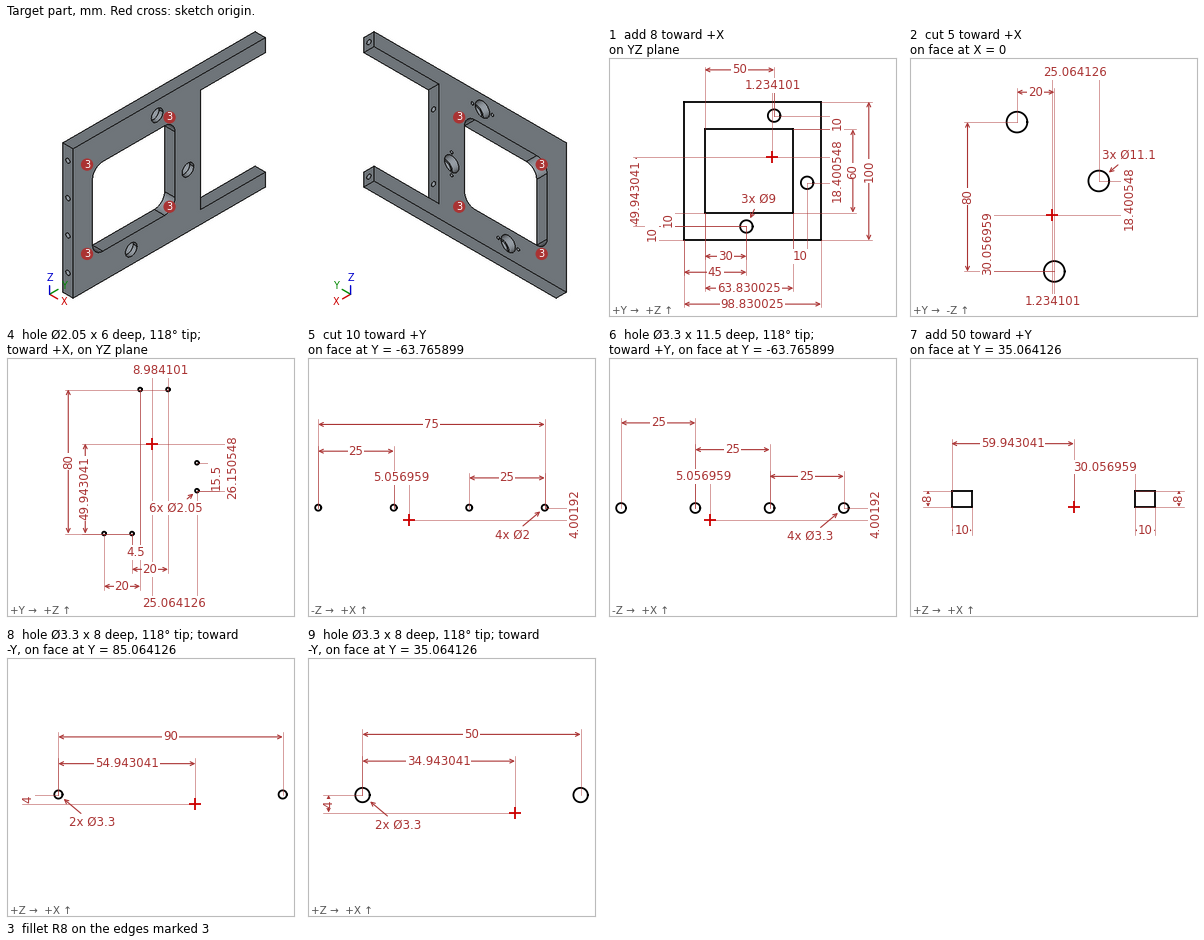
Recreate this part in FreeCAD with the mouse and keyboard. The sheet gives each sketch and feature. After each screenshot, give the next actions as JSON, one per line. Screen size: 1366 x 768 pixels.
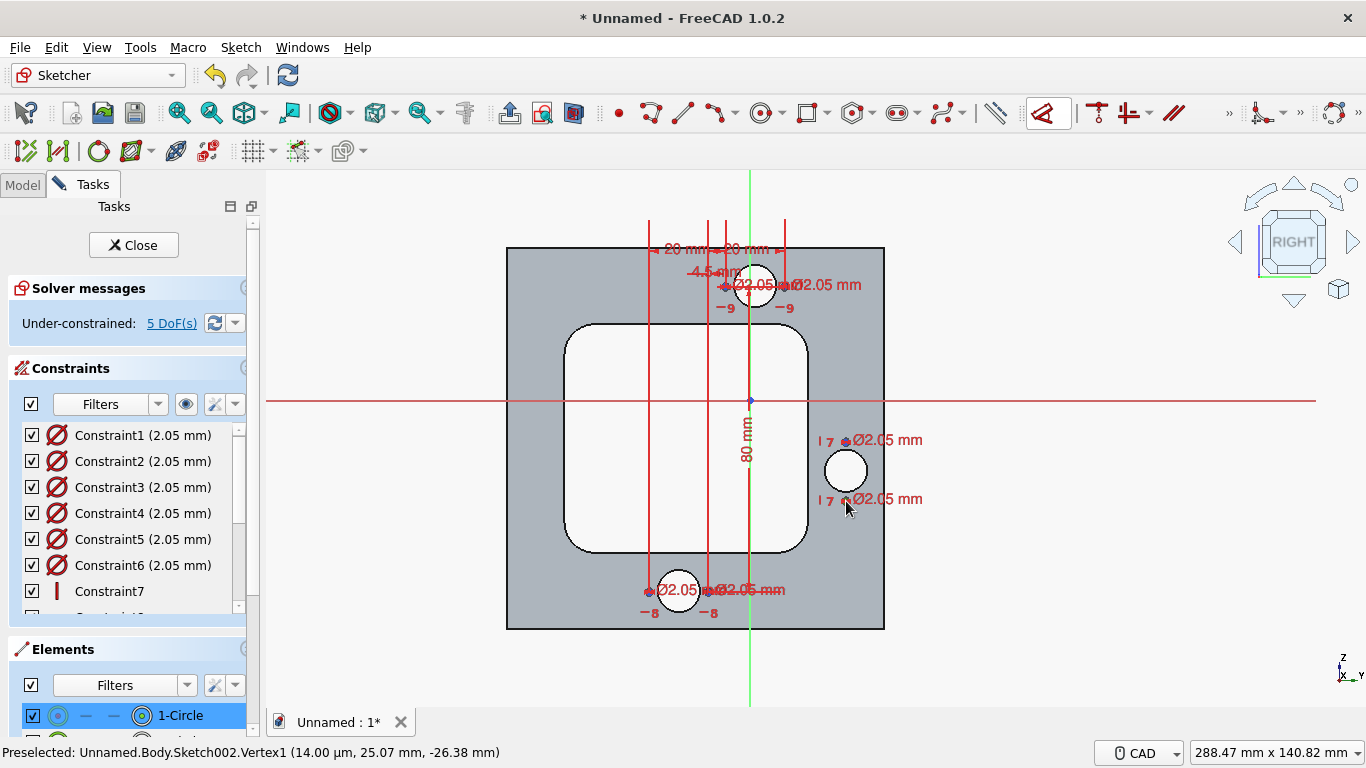
{"action": "left_click", "coordinate": [846, 442]}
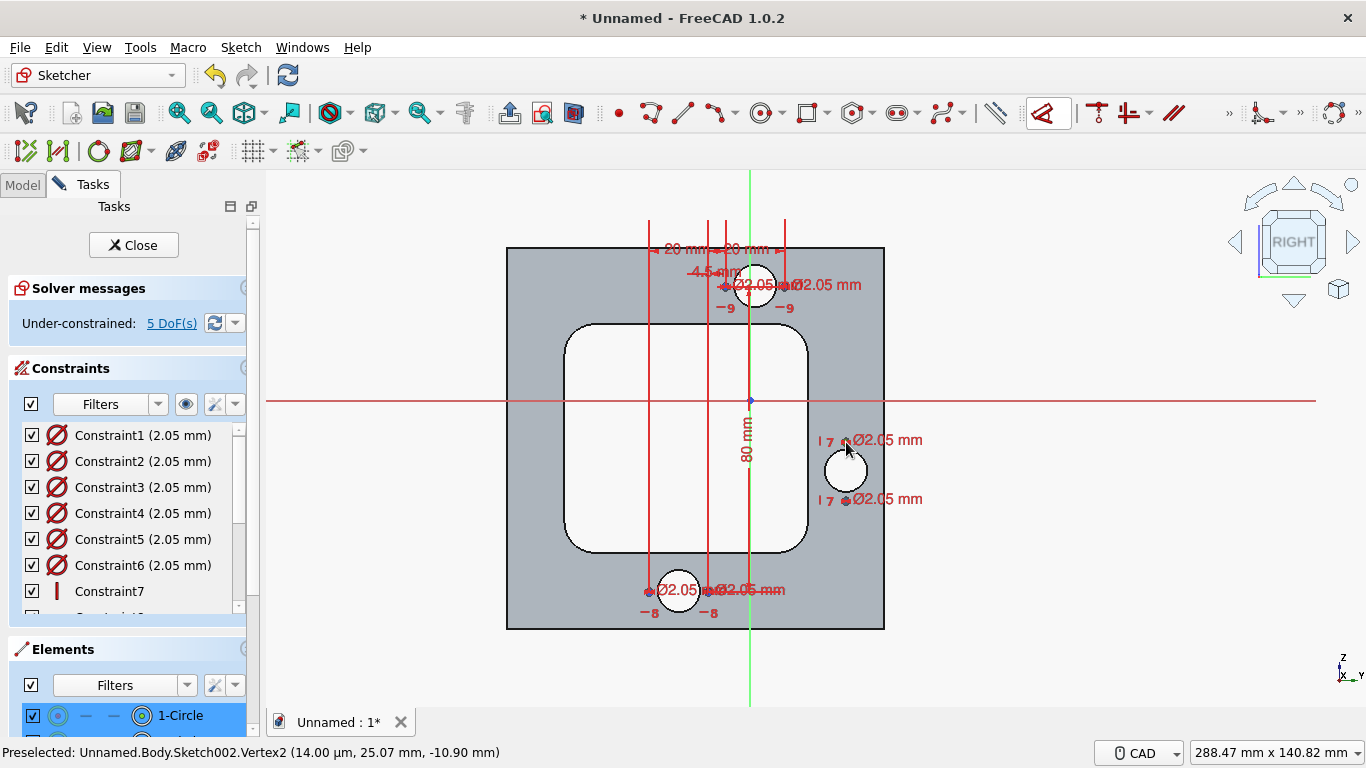
{"action": "key", "text": "i"}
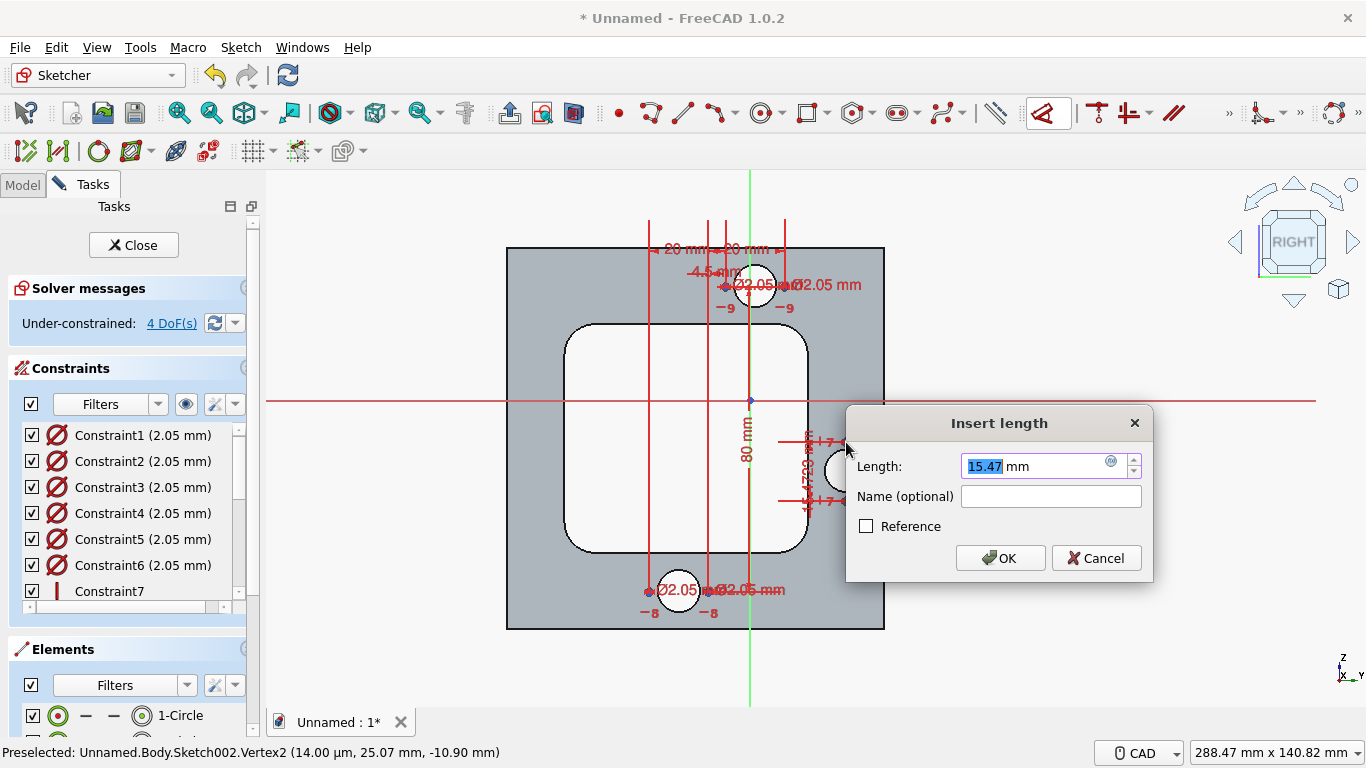
{"action": "type", "text": "15.5"}
{"action": "key", "text": "Return"}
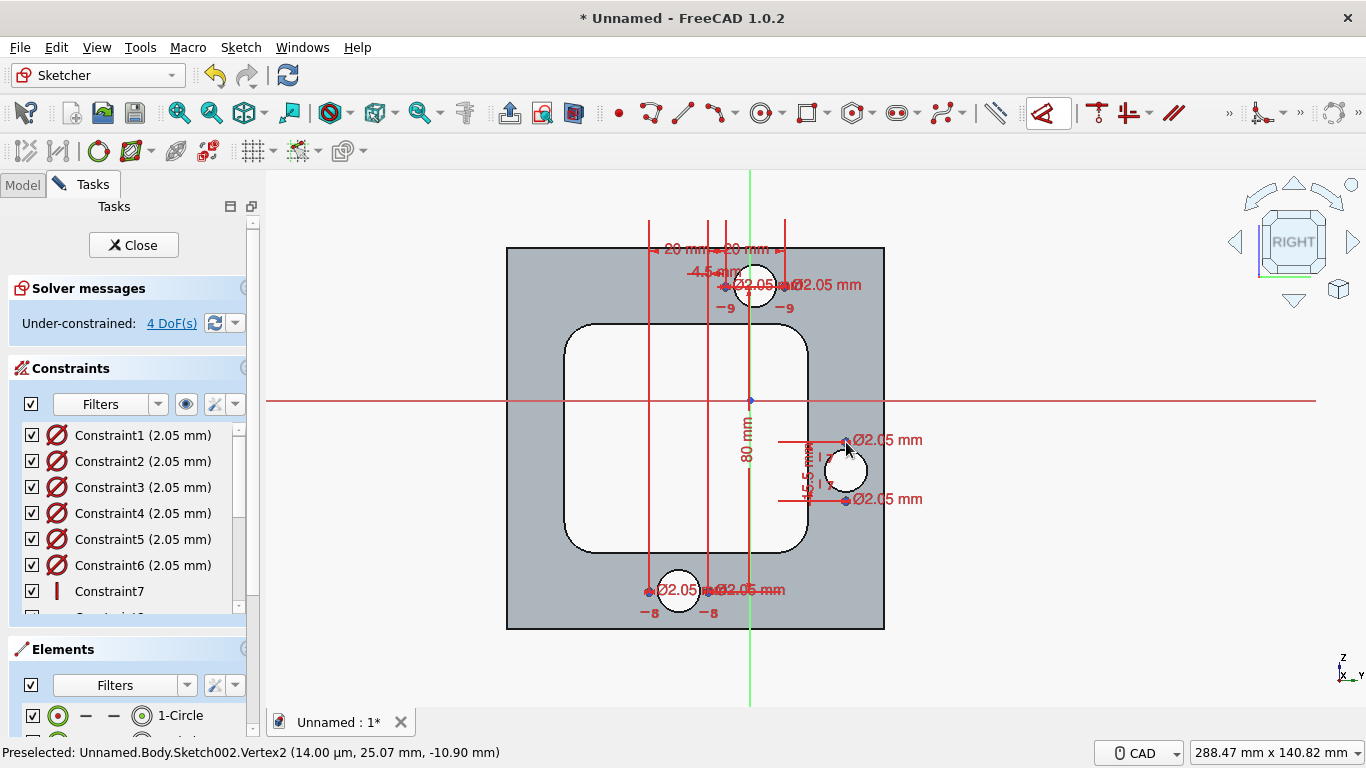
{"action": "left_click", "coordinate": [785, 287]}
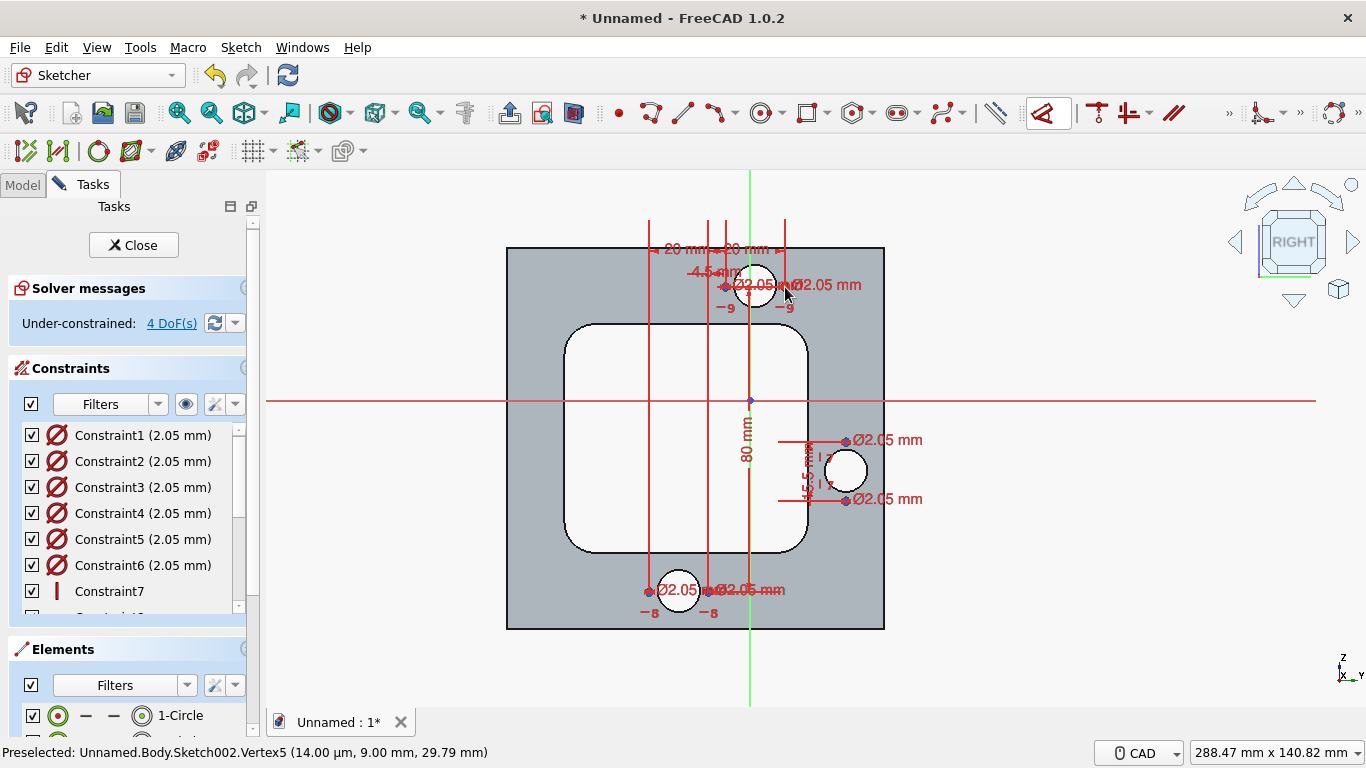
{"action": "left_click", "coordinate": [1066, 114]}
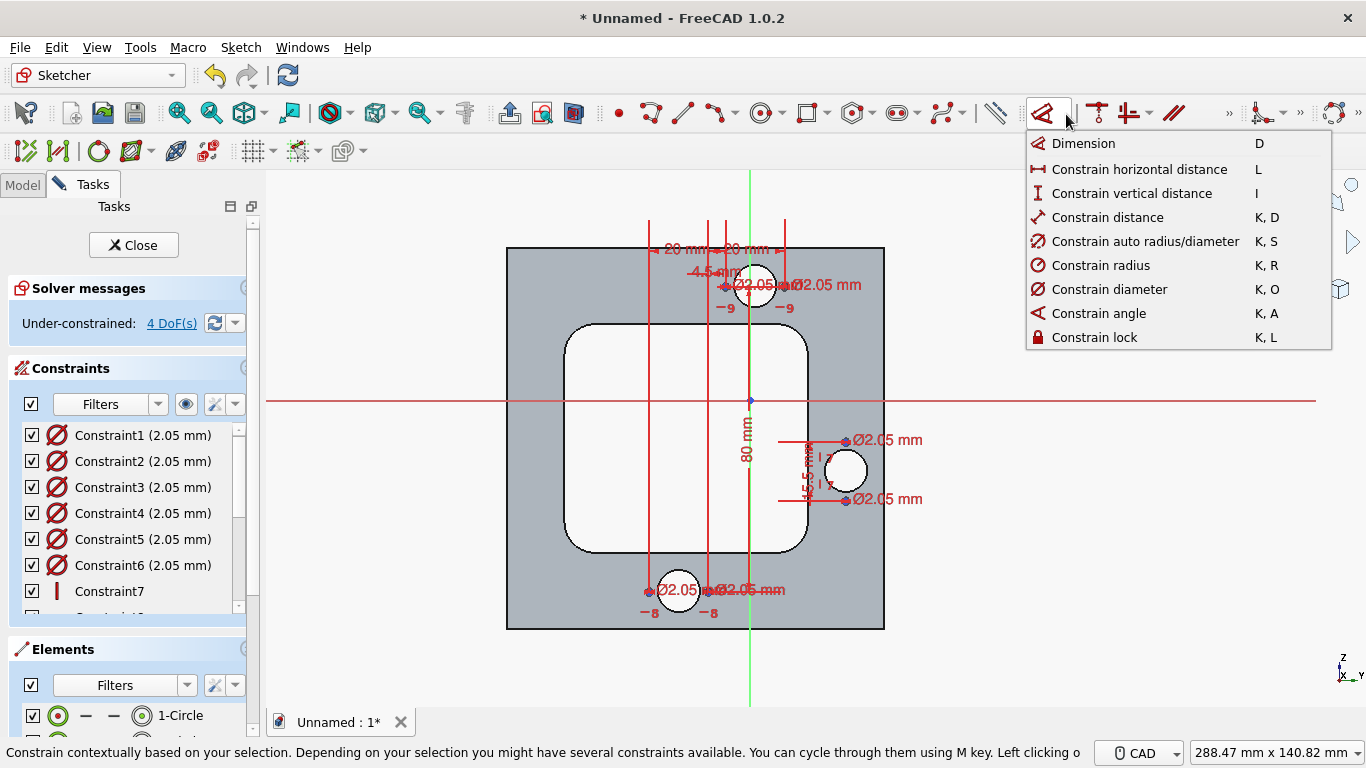
{"action": "left_click", "coordinate": [1179, 169]}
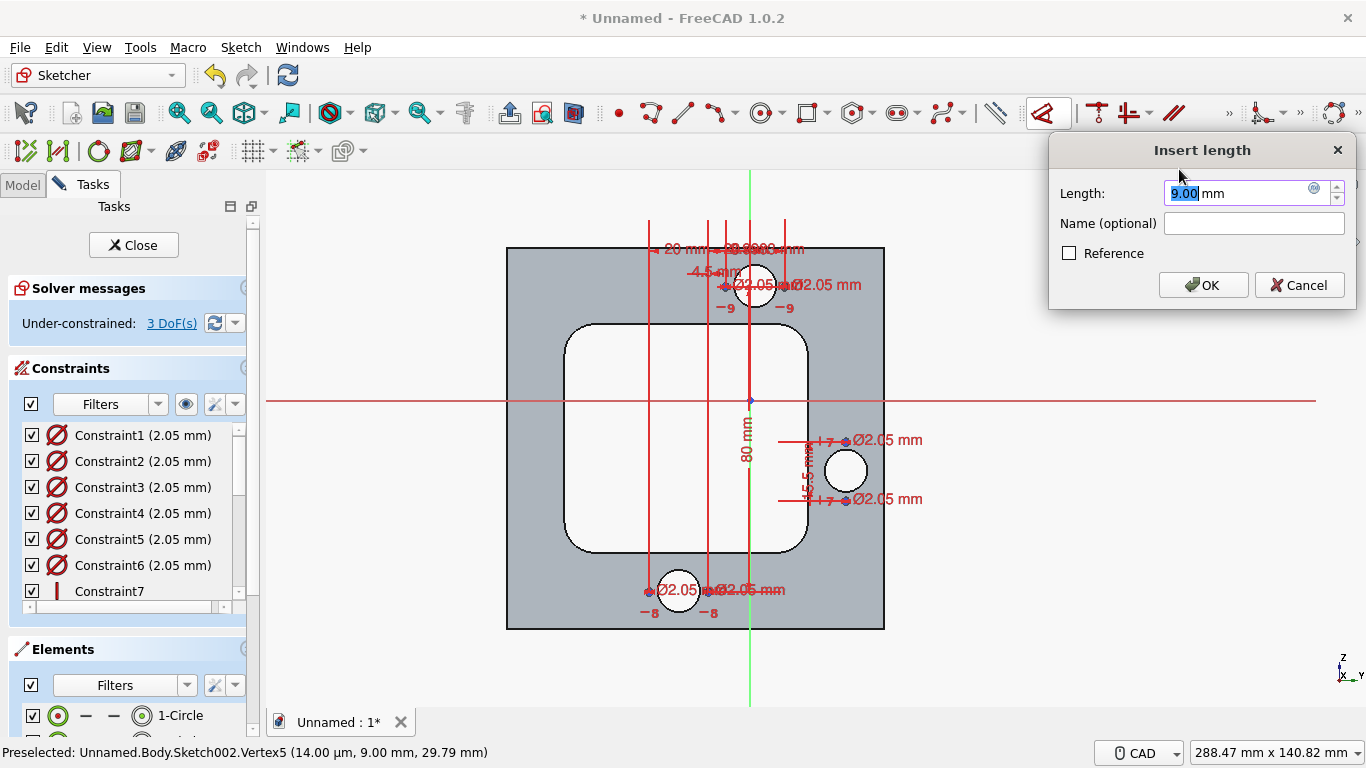
{"action": "type", "text": "8.984101"}
{"action": "key", "text": "Return"}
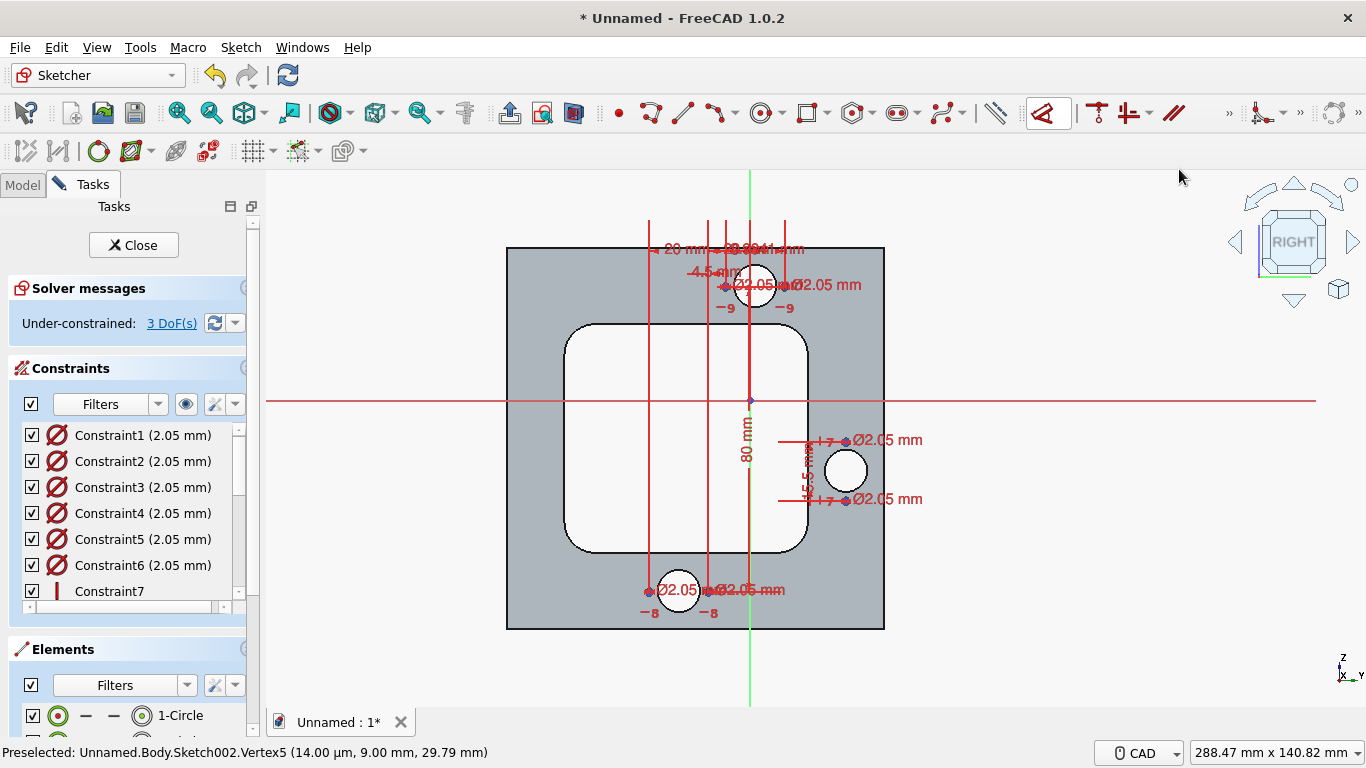
{"action": "left_click", "coordinate": [846, 501]}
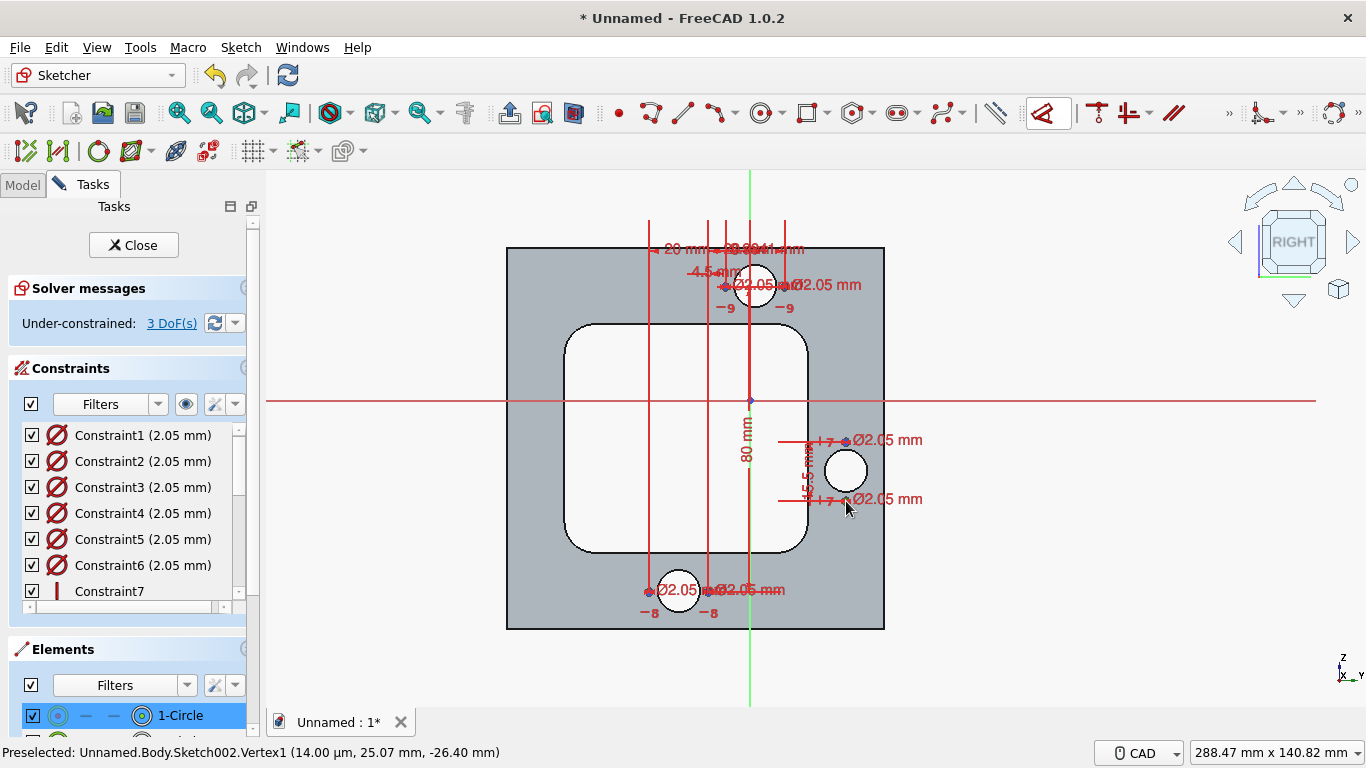
{"action": "left_click", "coordinate": [1066, 114]}